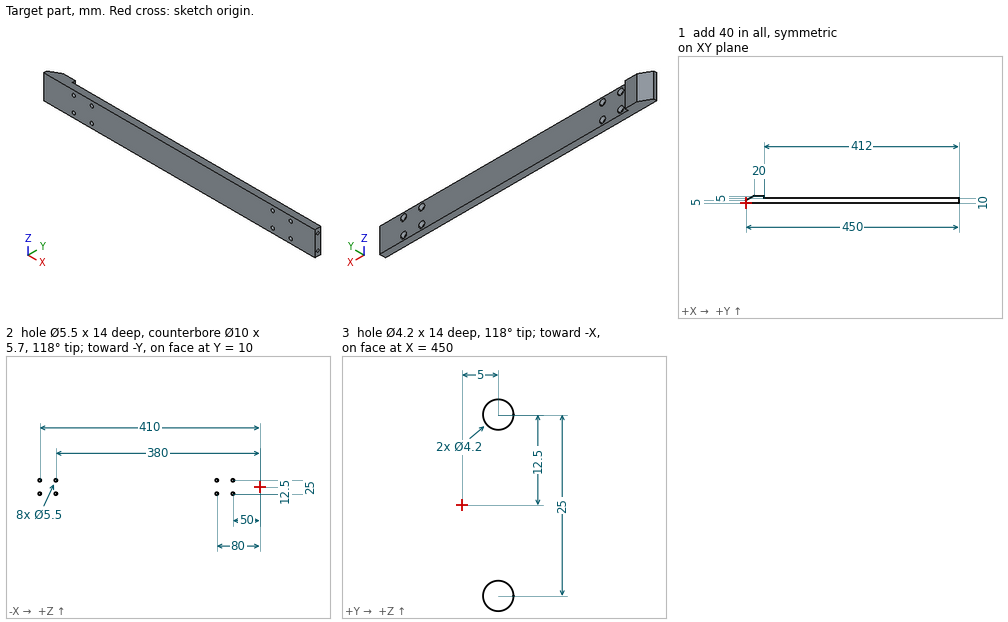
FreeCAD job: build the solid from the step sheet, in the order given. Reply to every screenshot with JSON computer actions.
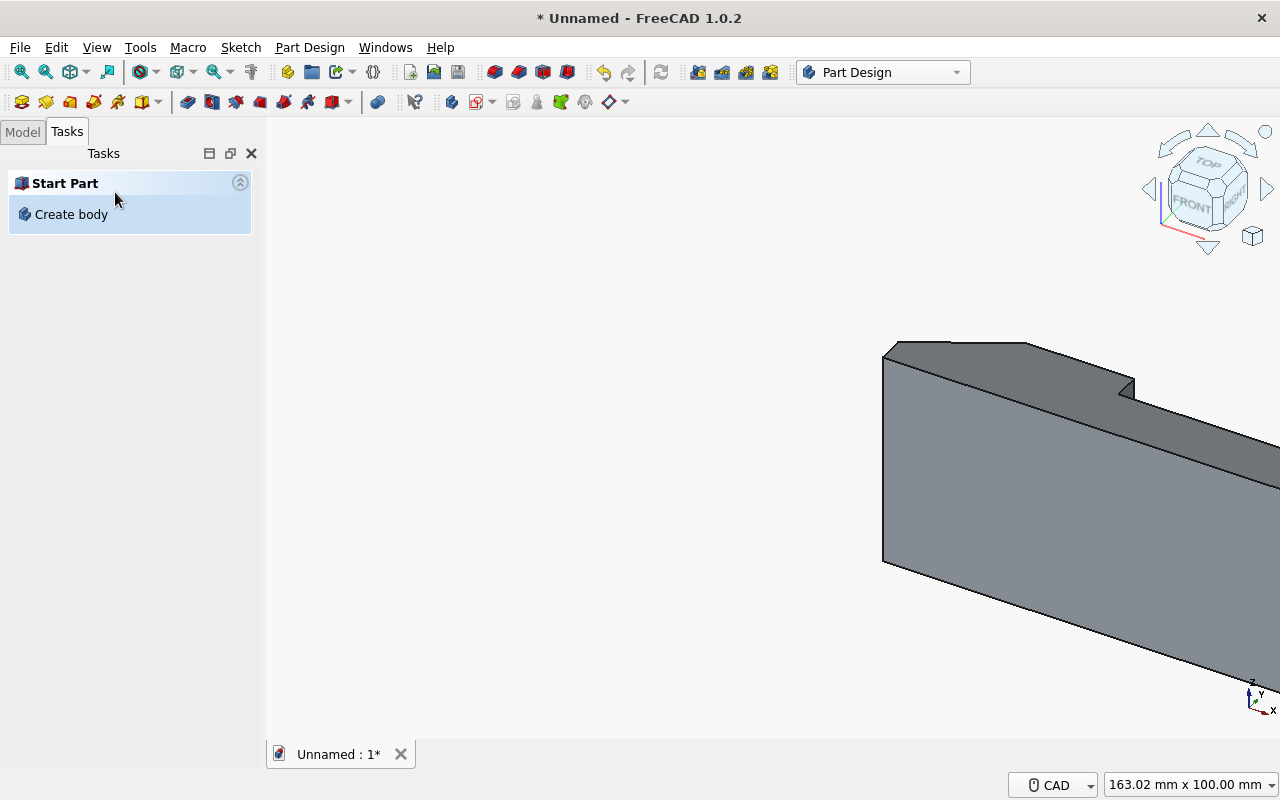
{"action": "left_click", "coordinate": [22, 72]}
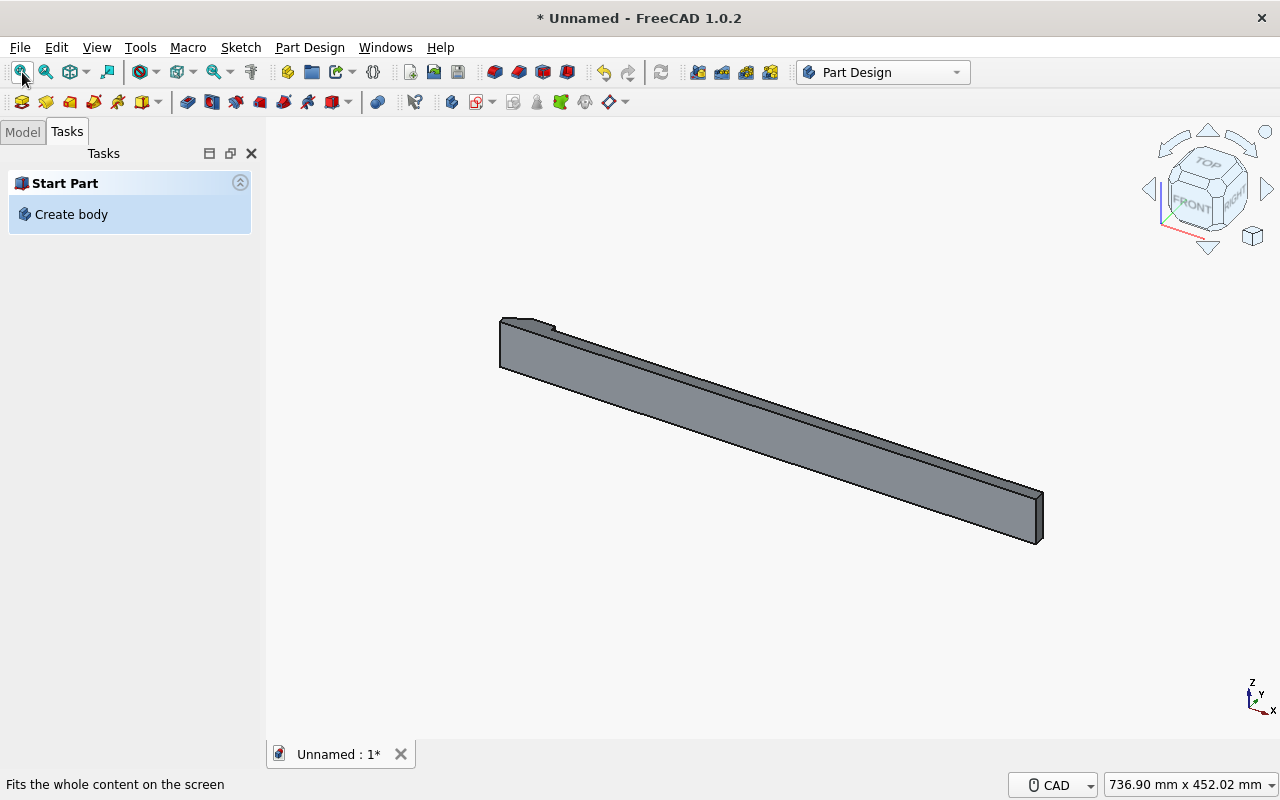
{"action": "key", "text": "4"}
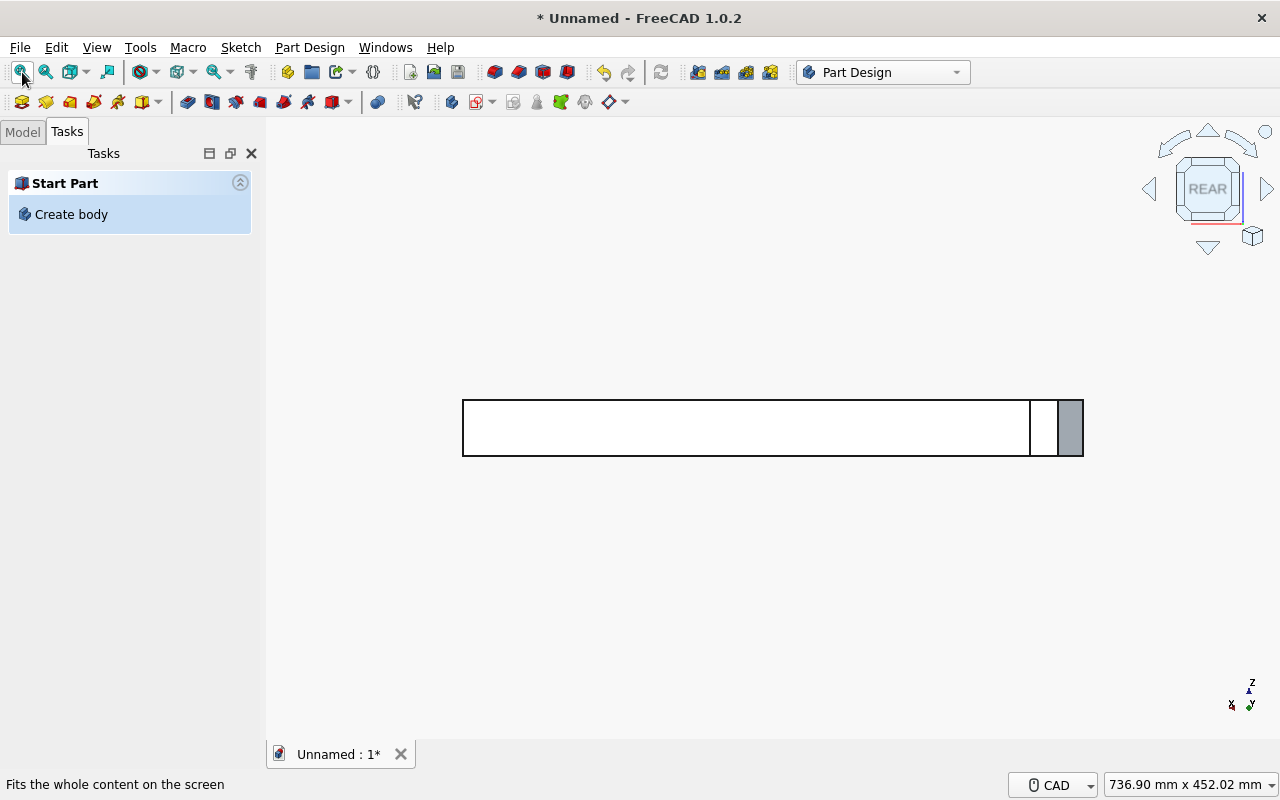
{"action": "left_click", "coordinate": [504, 427]}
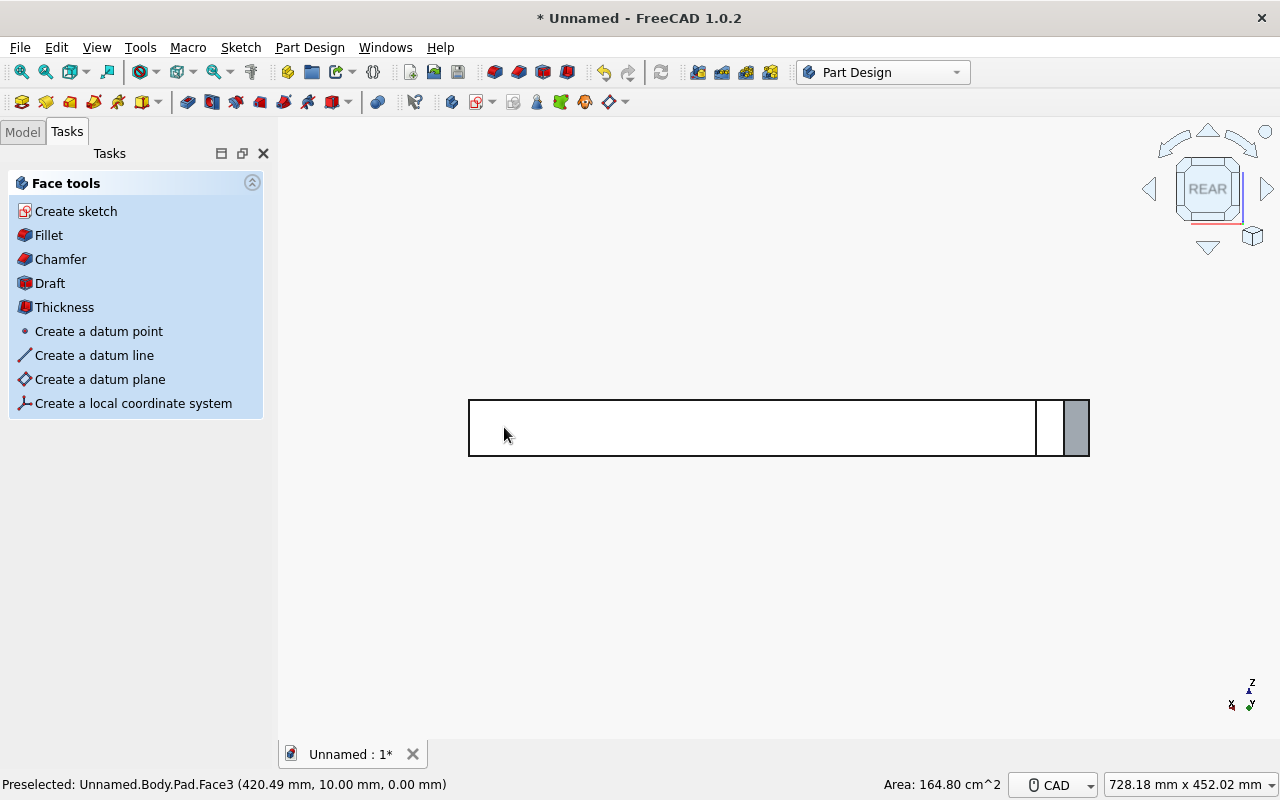
{"action": "left_click", "coordinate": [476, 102]}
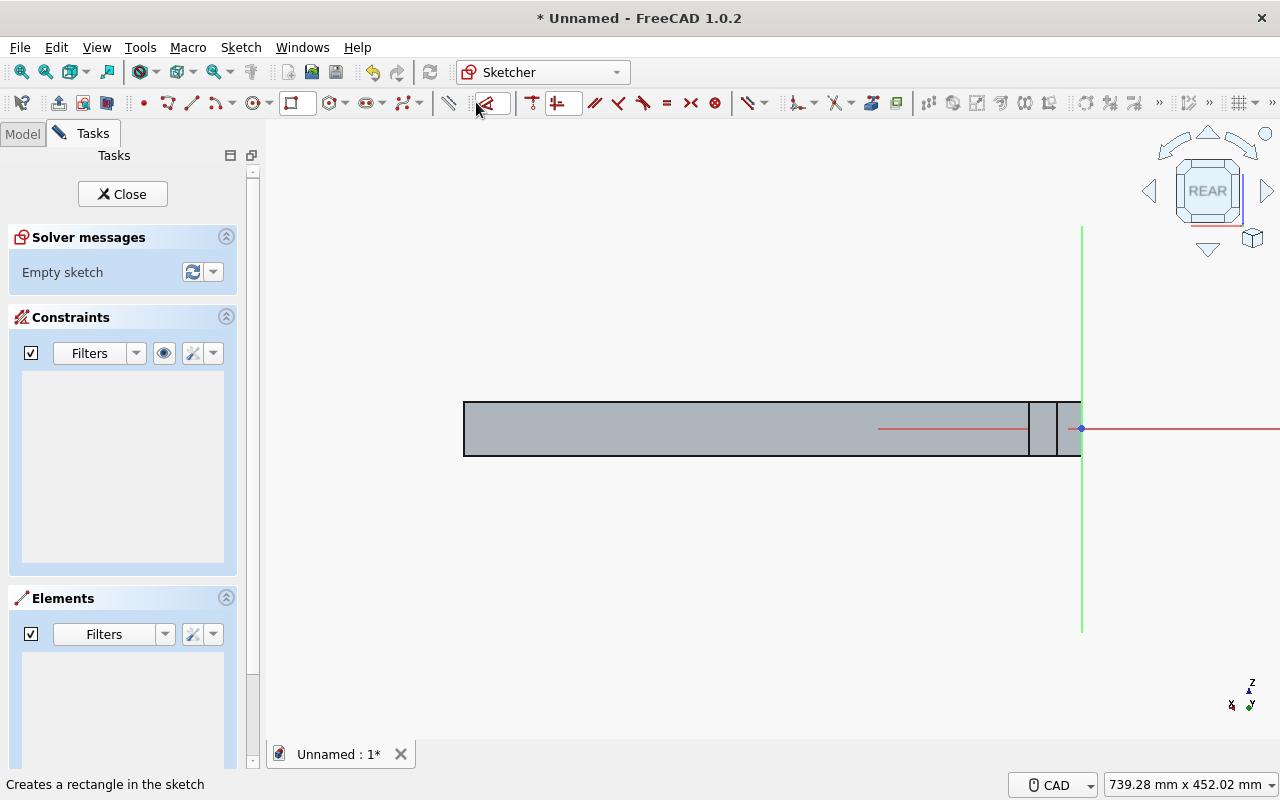
{"action": "key", "text": "q s"}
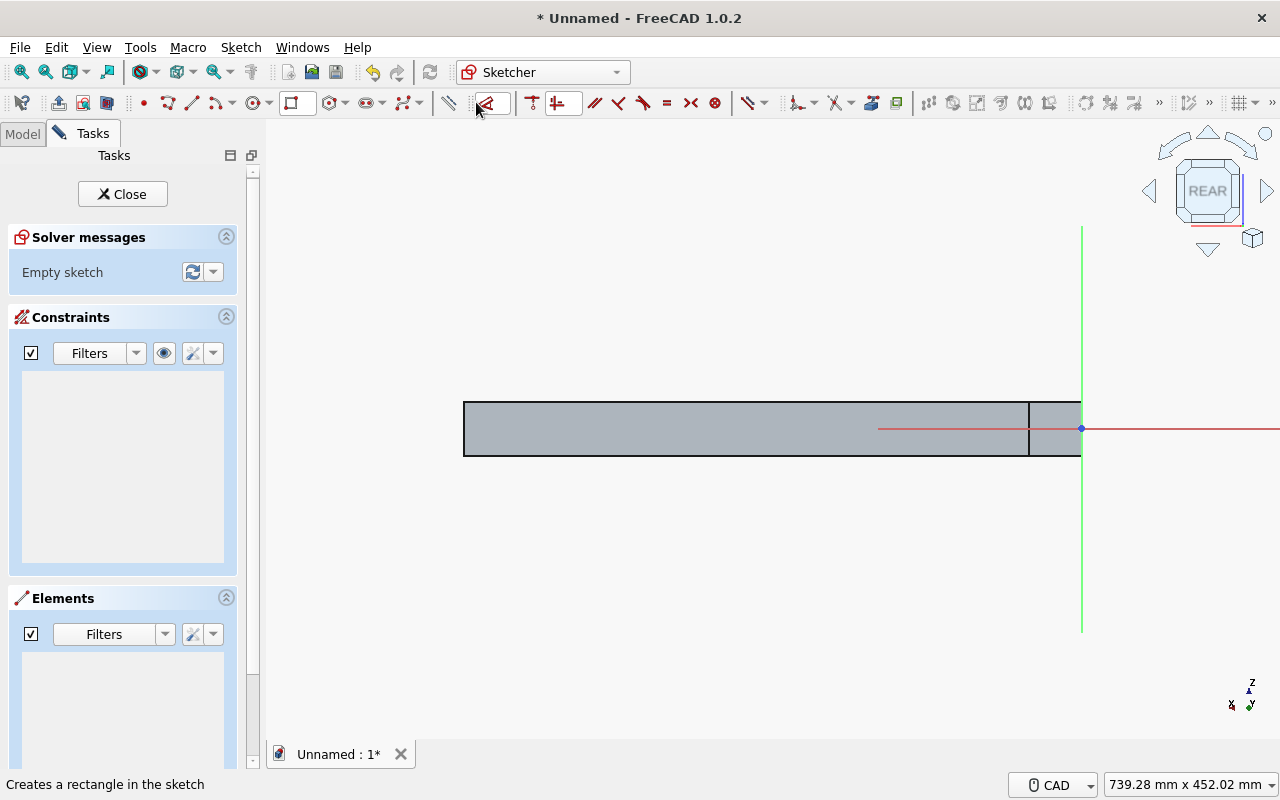
{"action": "left_click", "coordinate": [254, 104]}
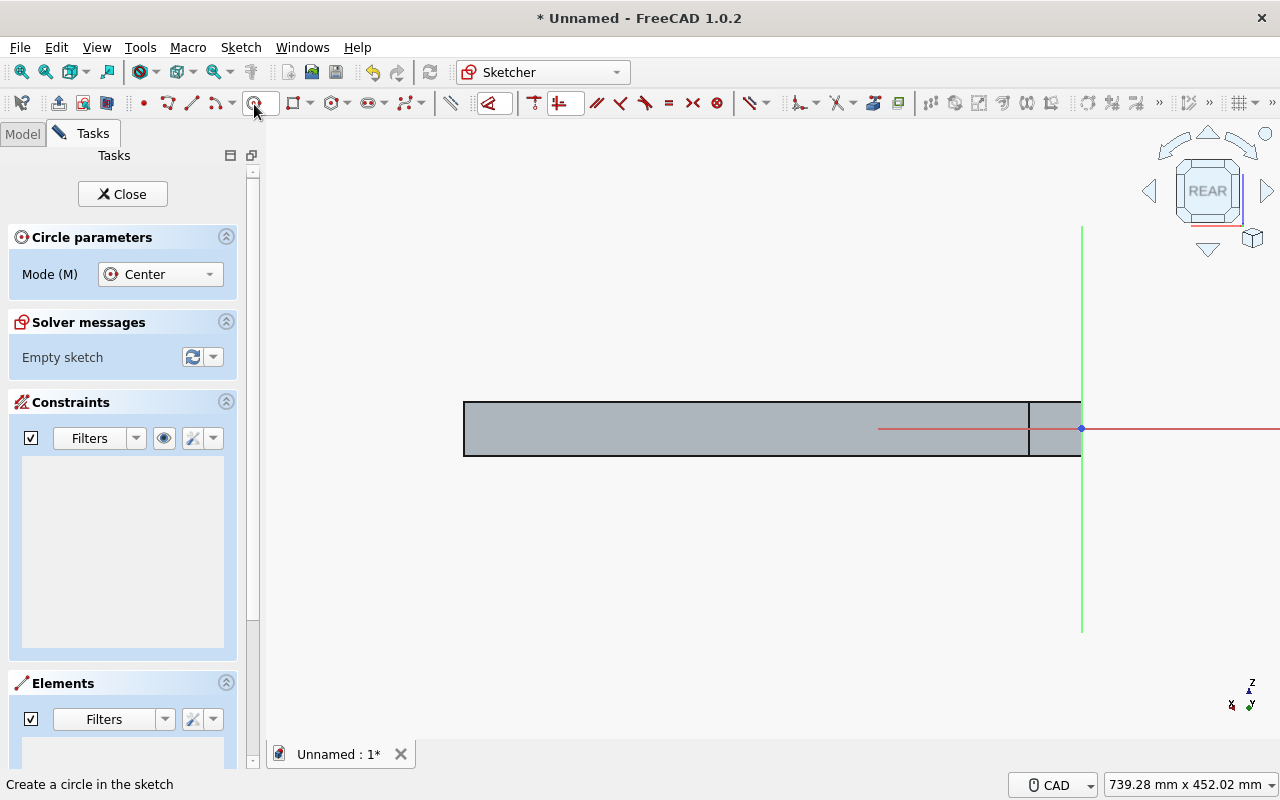
{"action": "scroll", "coordinate": [1013, 446], "scroll_direction": "up", "scroll_amount": 9}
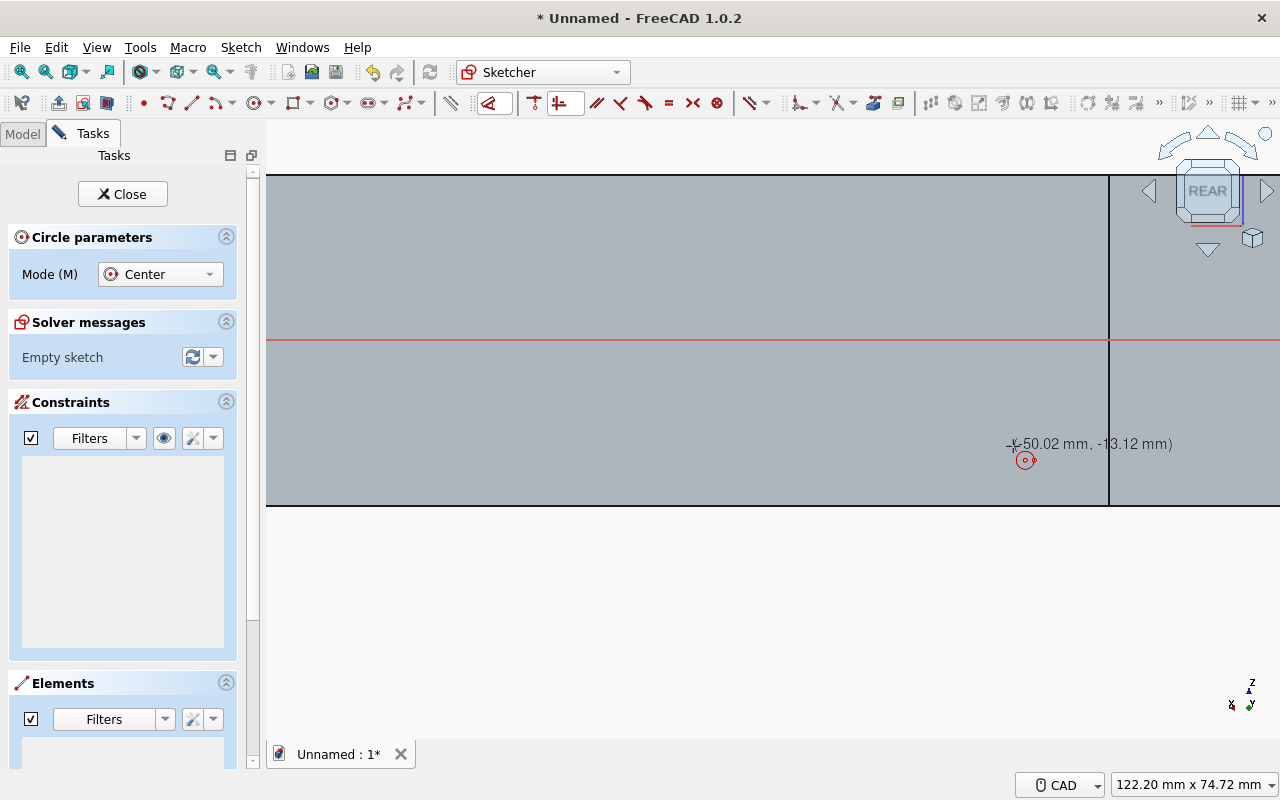
{"action": "scroll", "coordinate": [901, 447], "scroll_direction": "down", "scroll_amount": 9}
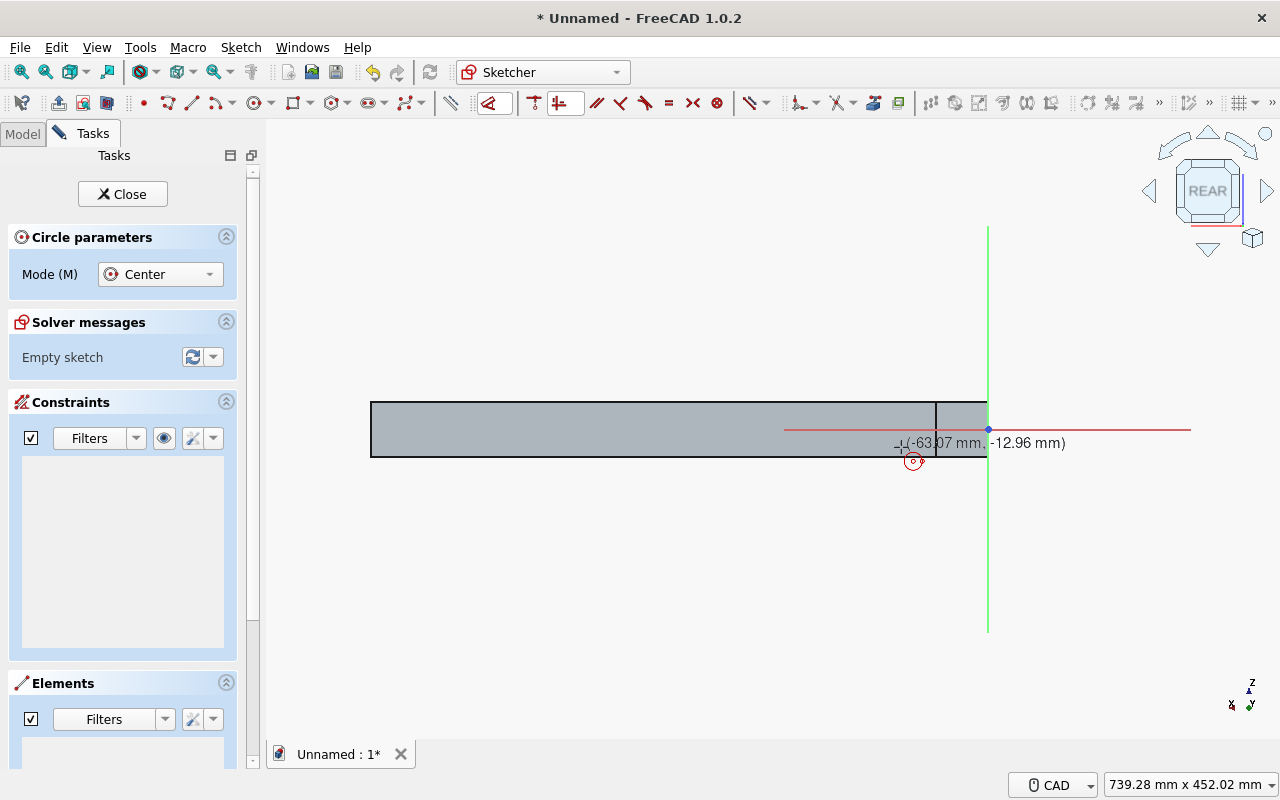
{"action": "left_click", "coordinate": [919, 447]}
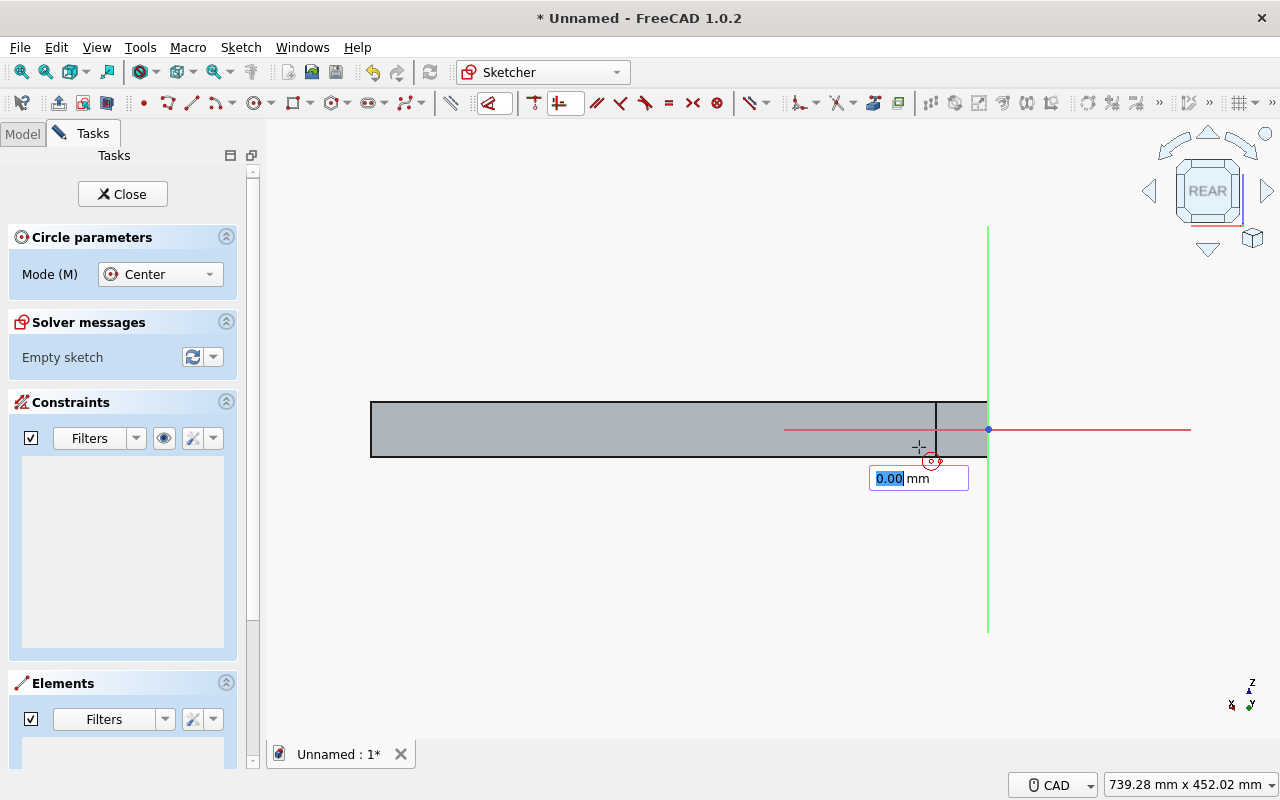
{"action": "scroll", "coordinate": [922, 444], "scroll_direction": "up", "scroll_amount": 8}